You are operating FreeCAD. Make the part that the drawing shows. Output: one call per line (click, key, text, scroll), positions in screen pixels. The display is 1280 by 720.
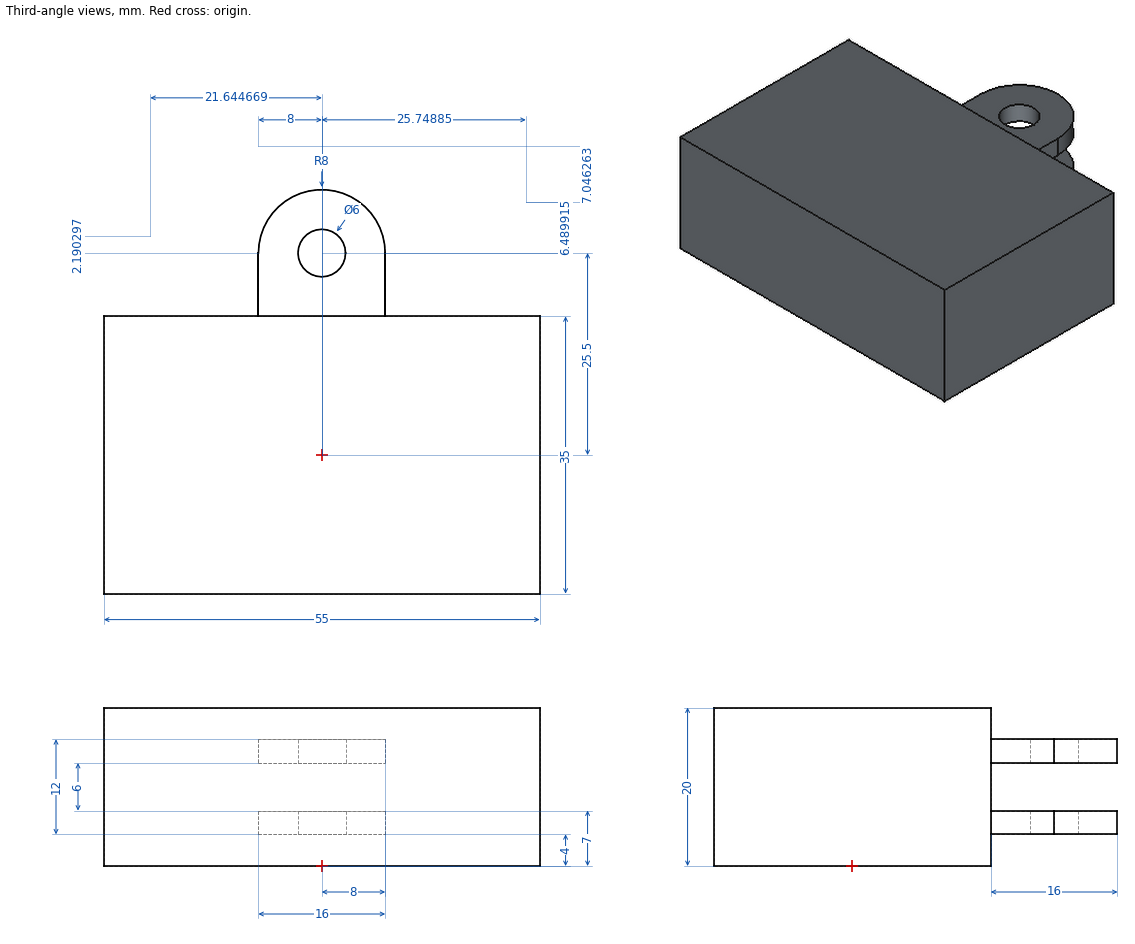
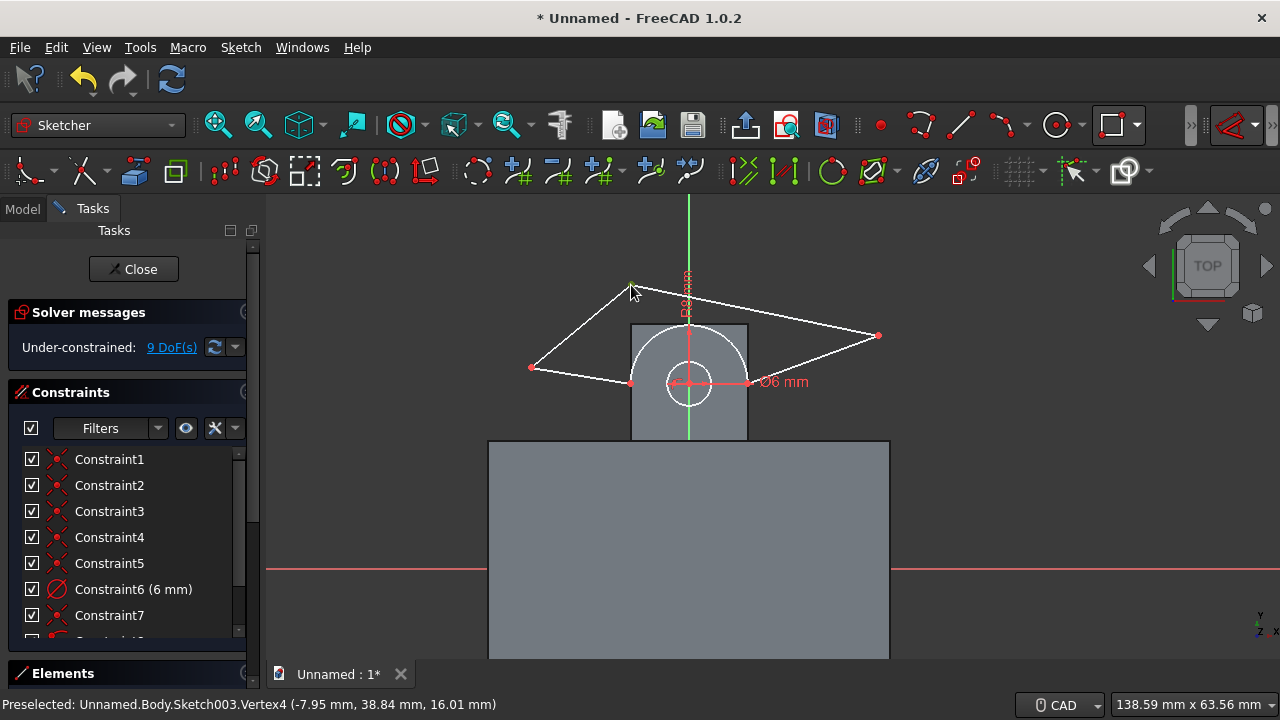
click(1258, 126)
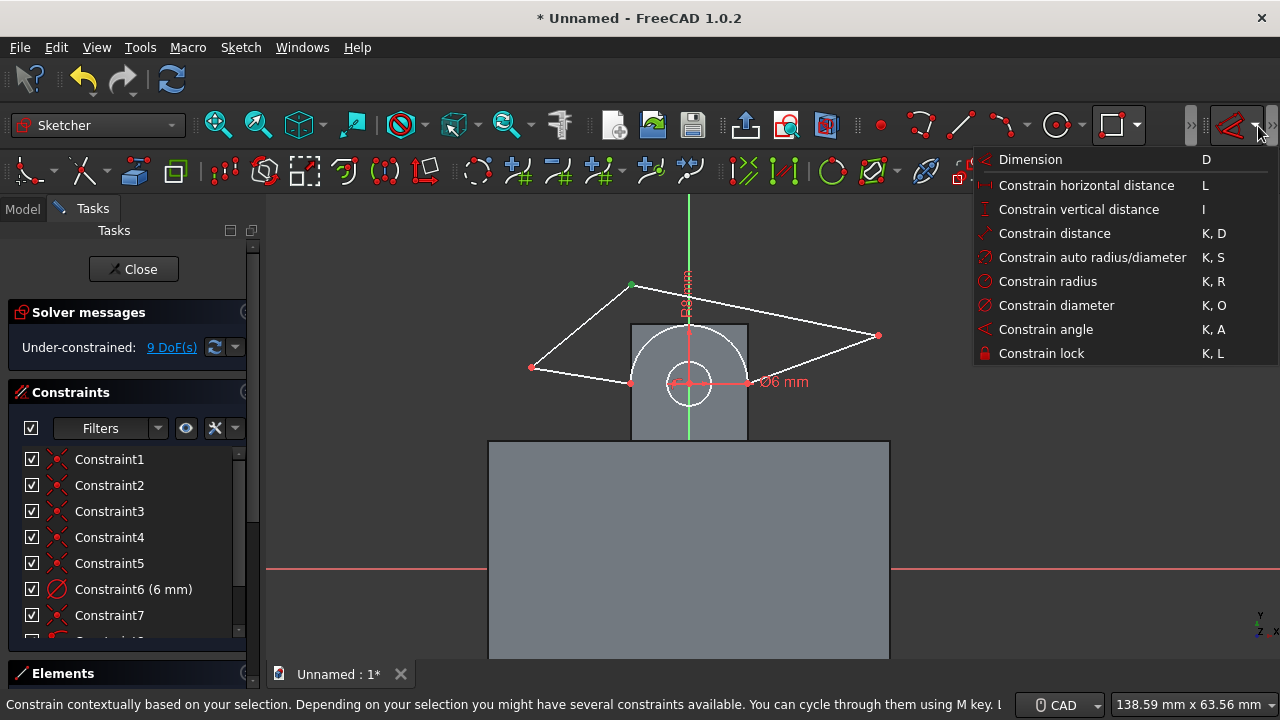
click(1126, 185)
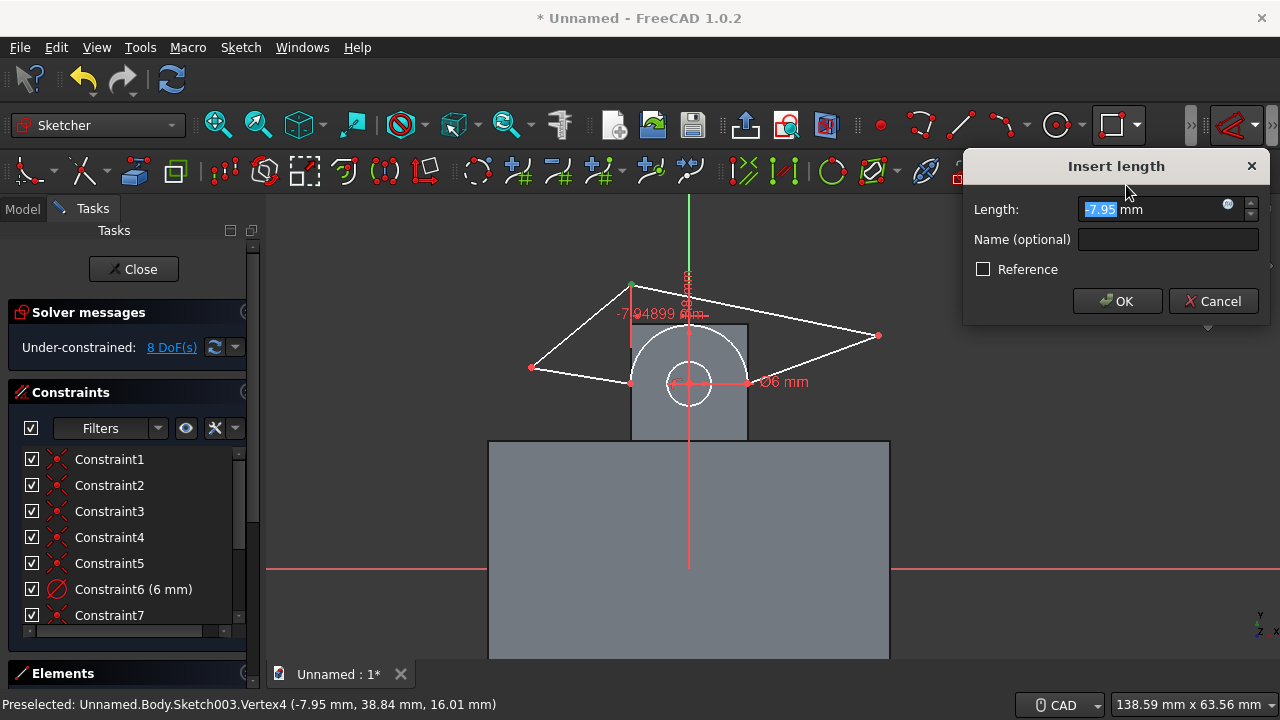
text(-8)
key(Return)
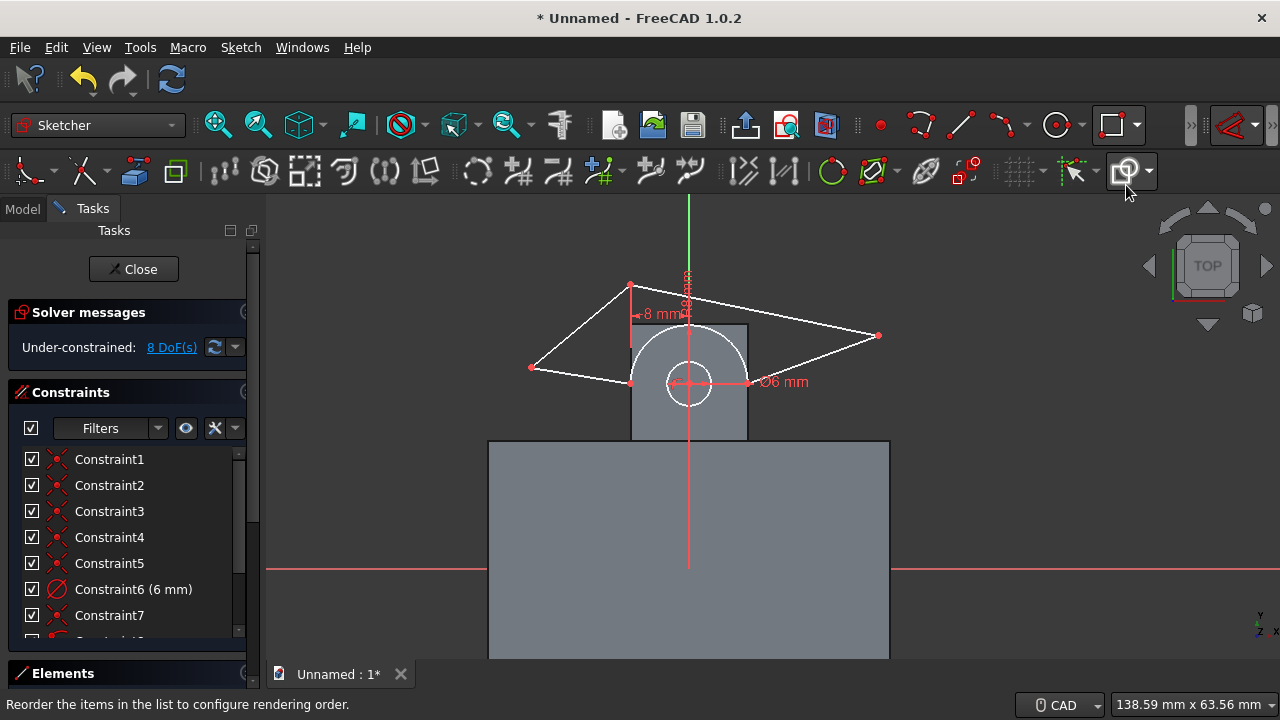
click(689, 384)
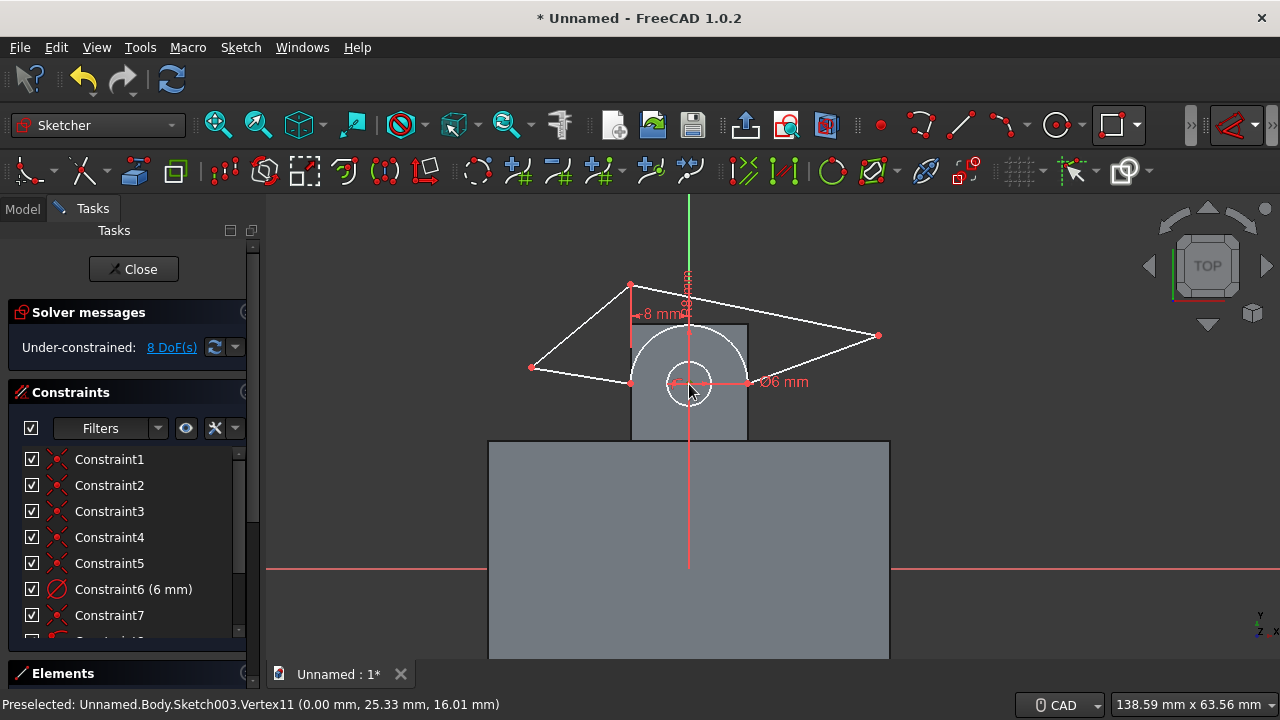
key(i)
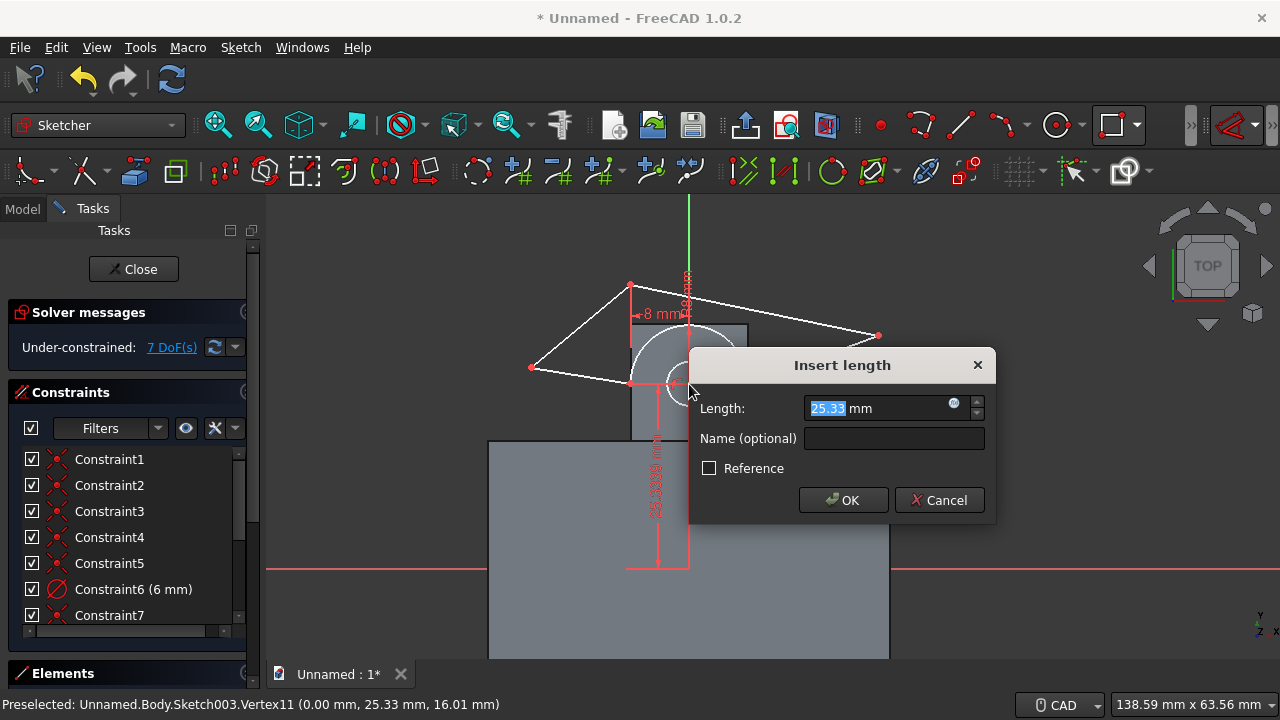
text(25.5)
key(Return)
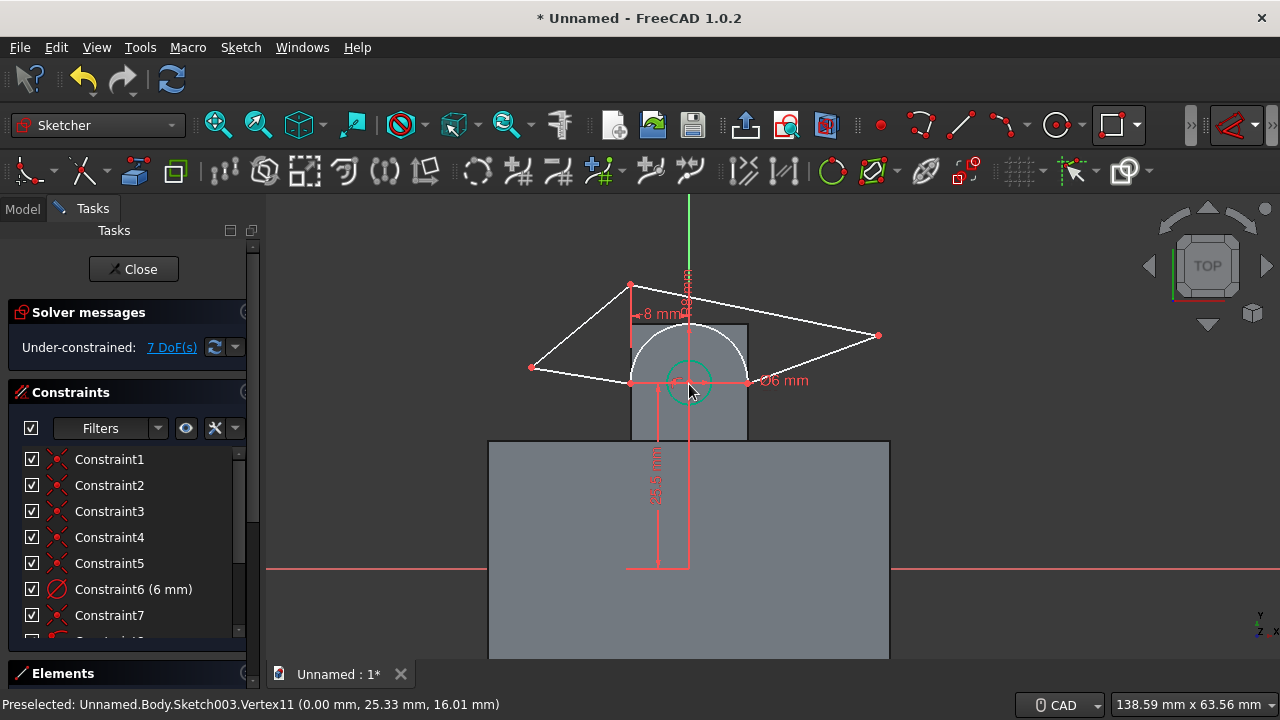
click(748, 384)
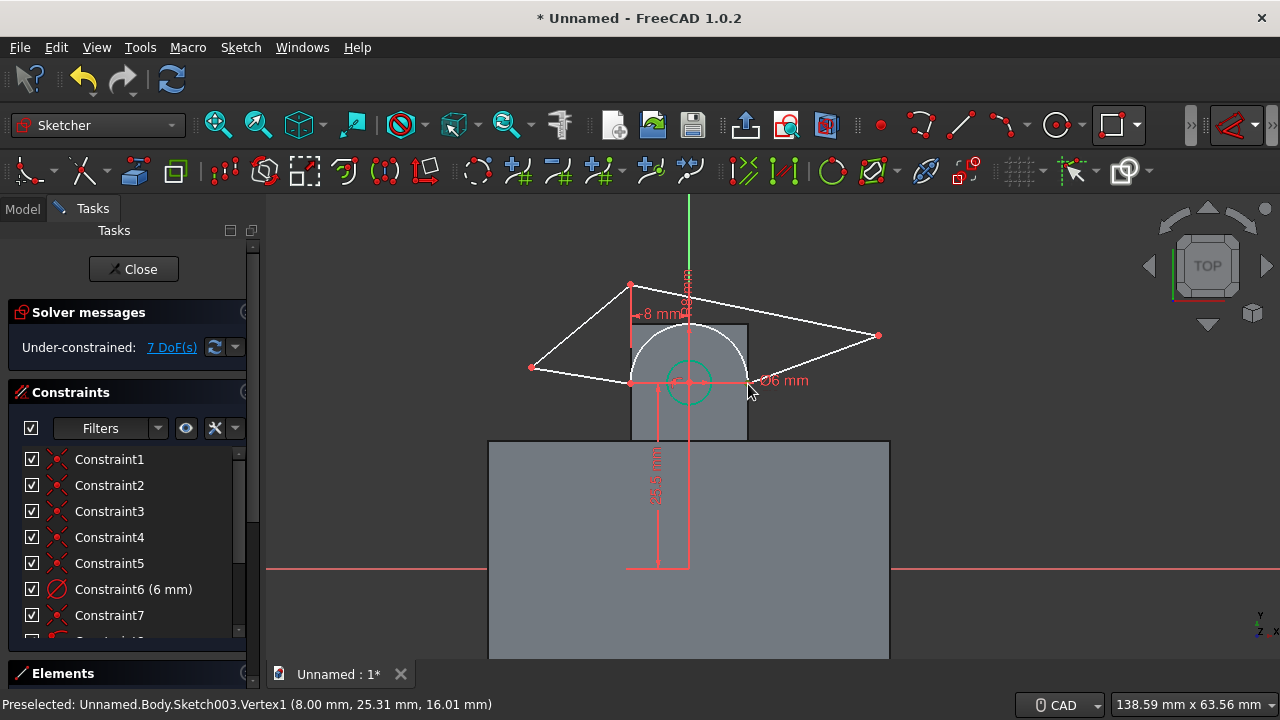
click(1258, 126)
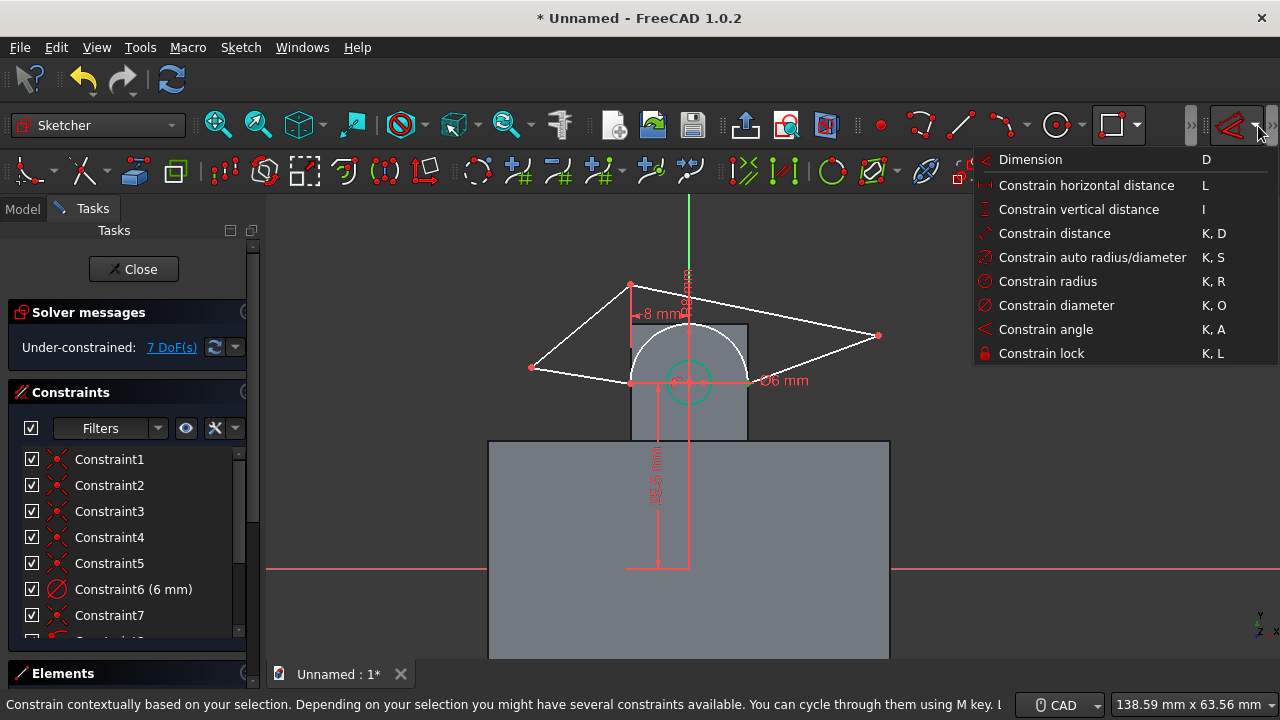
click(1126, 209)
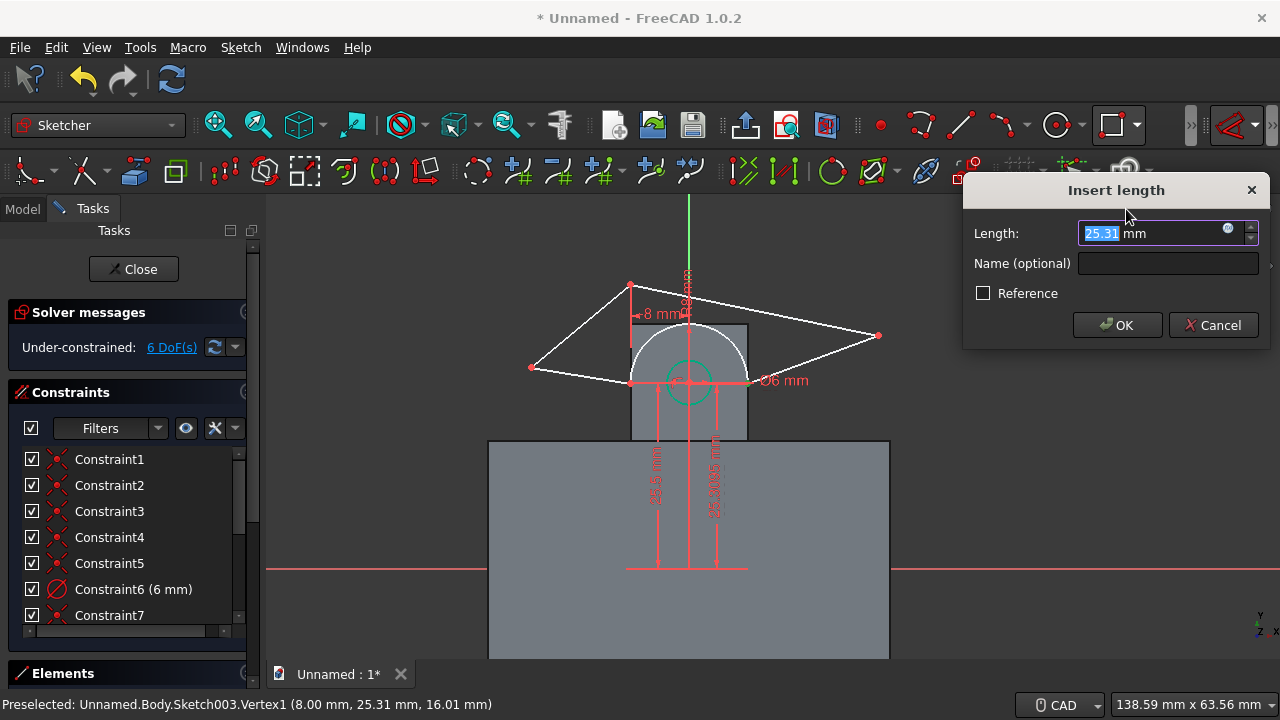
text(25.5)
key(Return)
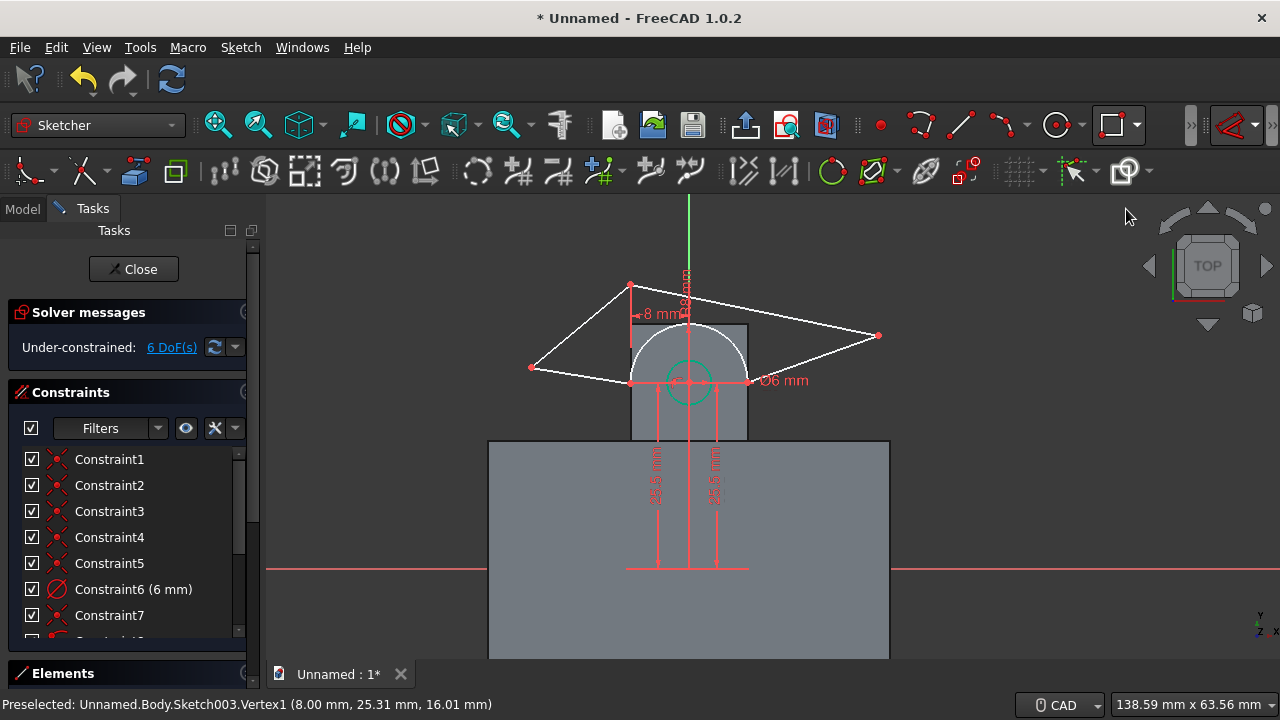
click(631, 384)